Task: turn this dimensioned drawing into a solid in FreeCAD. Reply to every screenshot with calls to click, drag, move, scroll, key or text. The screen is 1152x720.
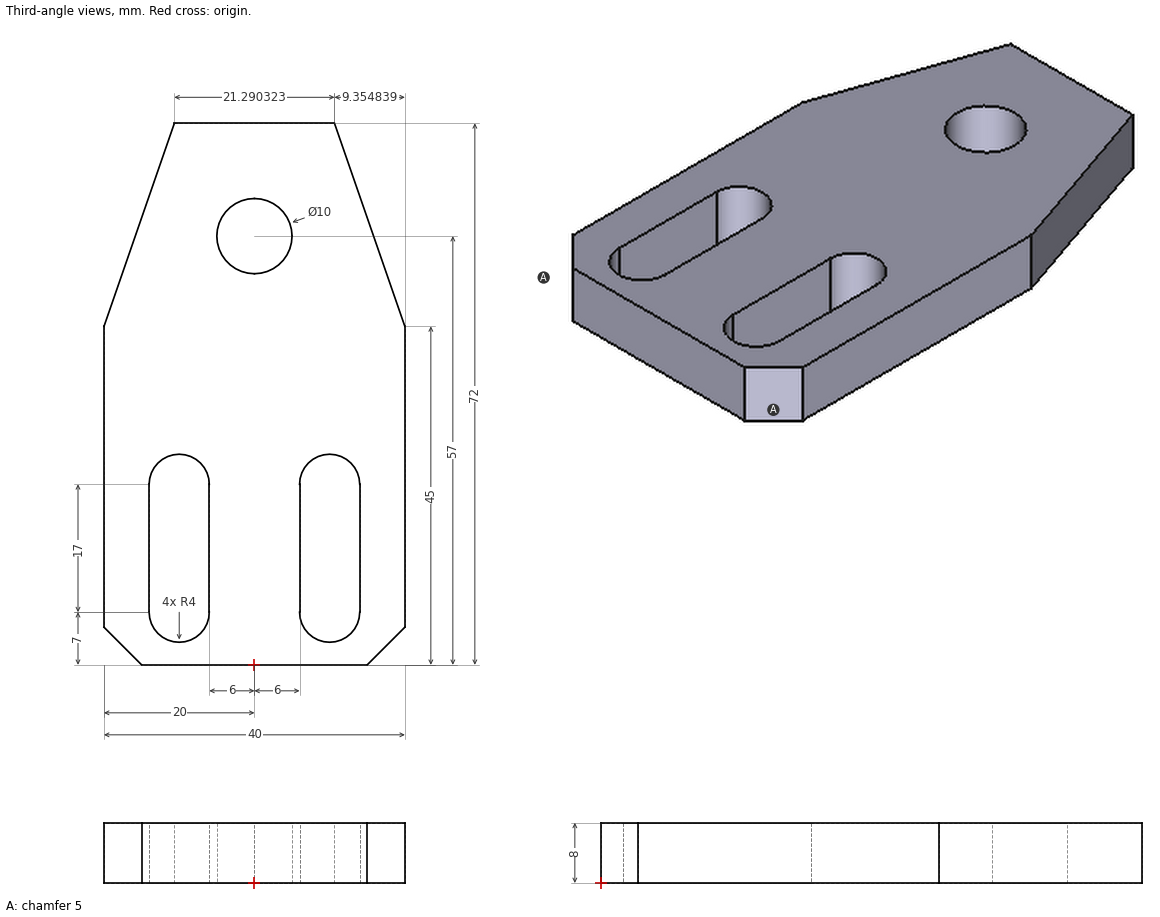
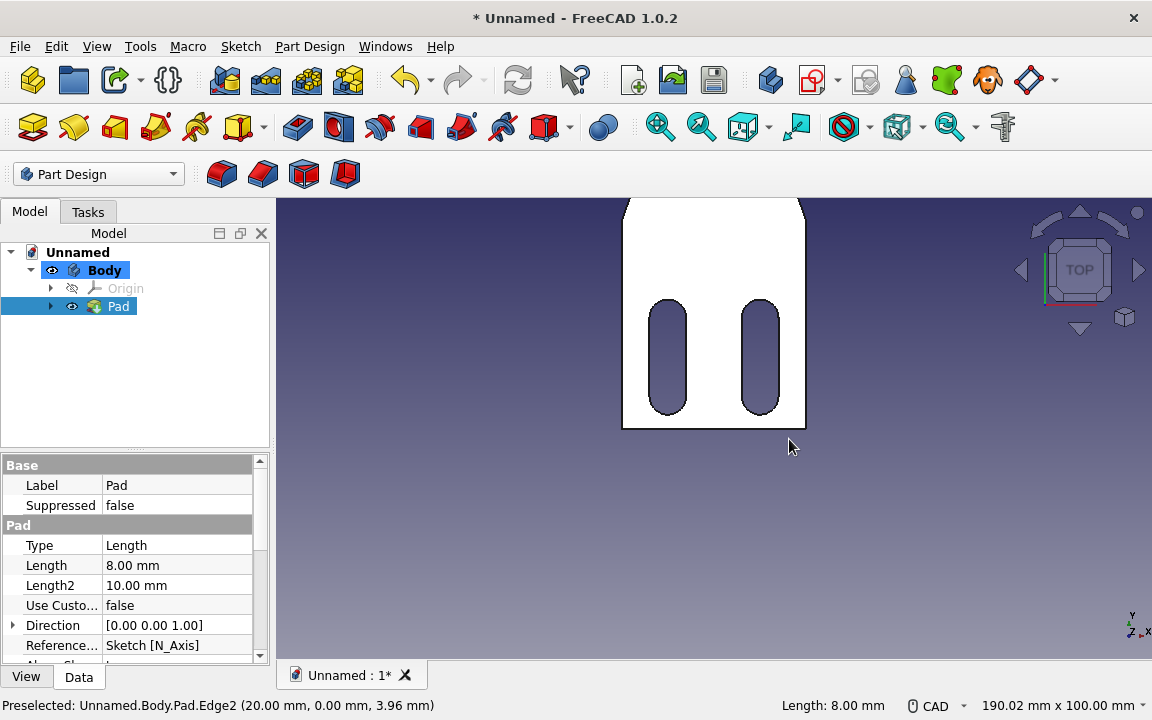
click(661, 128)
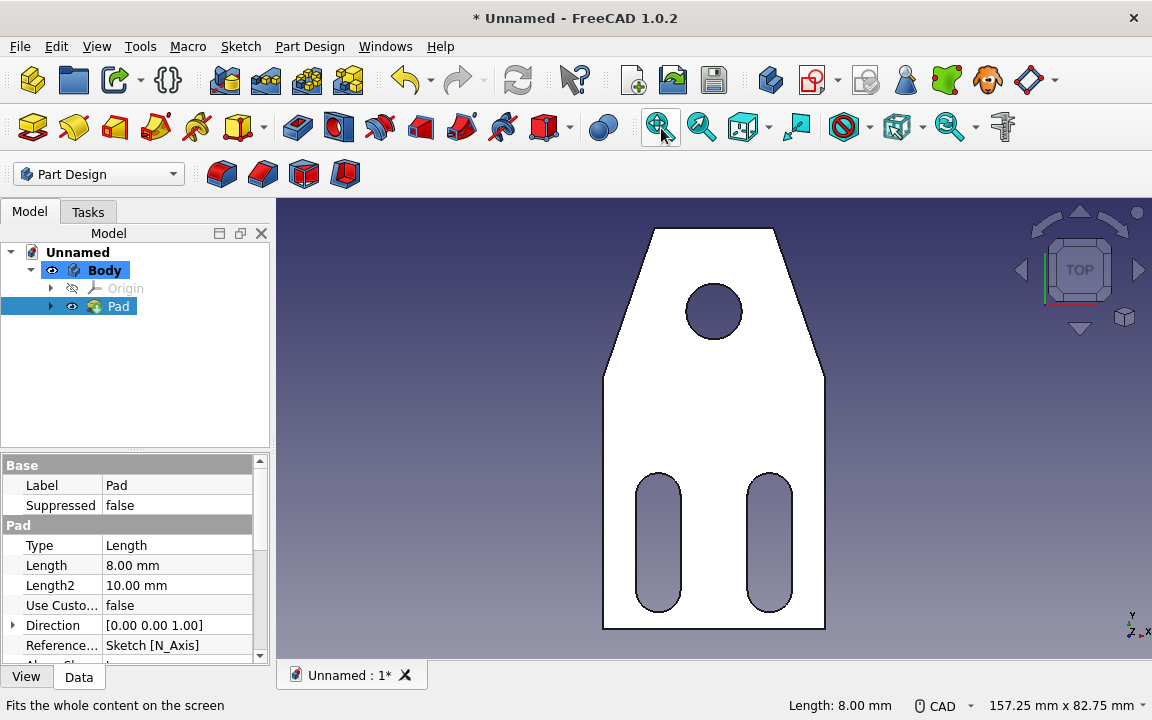
key(1)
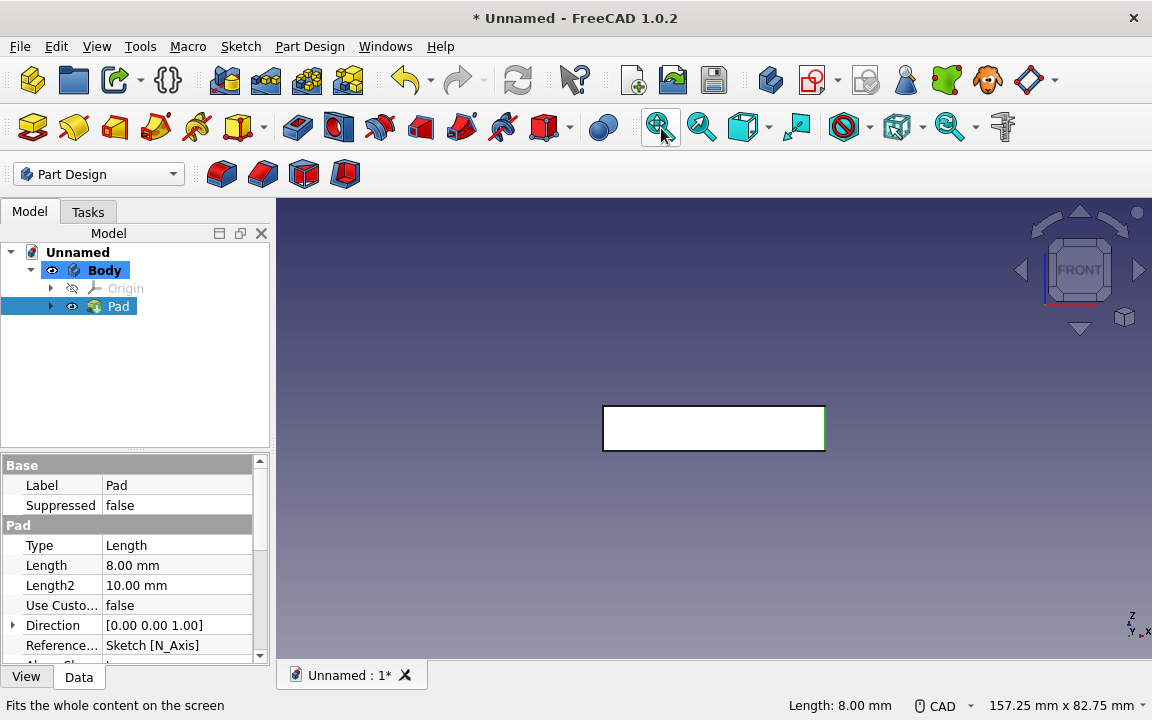
click(661, 128)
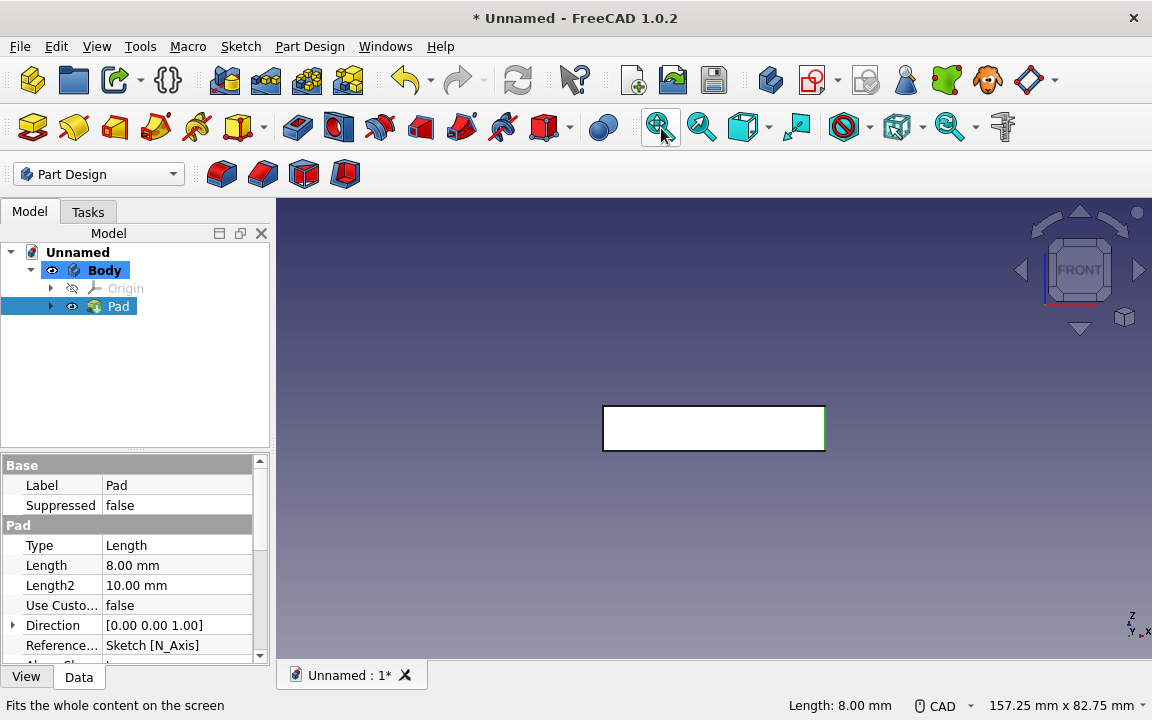
click(603, 428, ctrl)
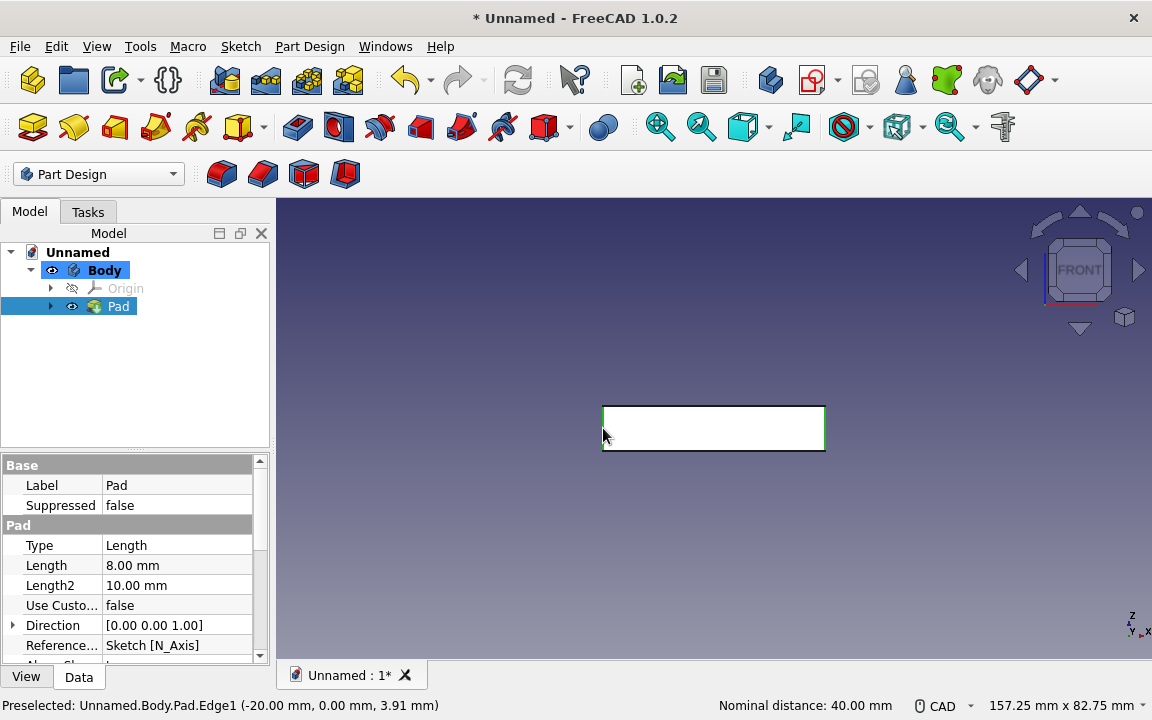
click(263, 174)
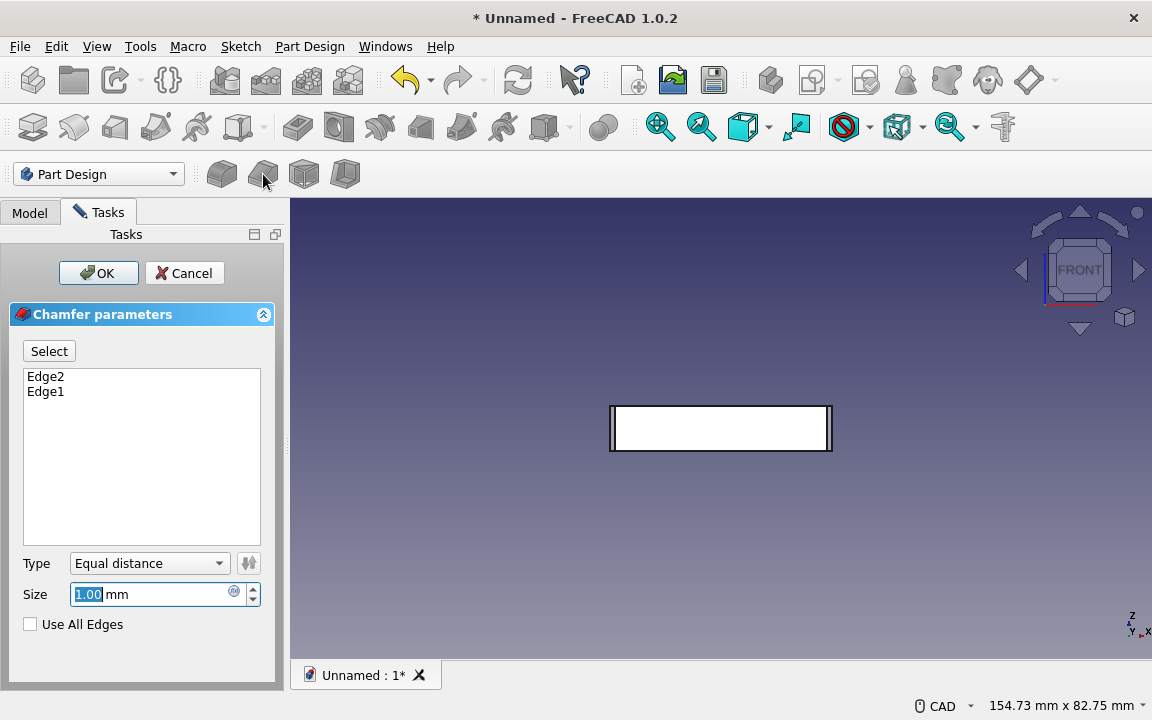
text(5)
key(Tab)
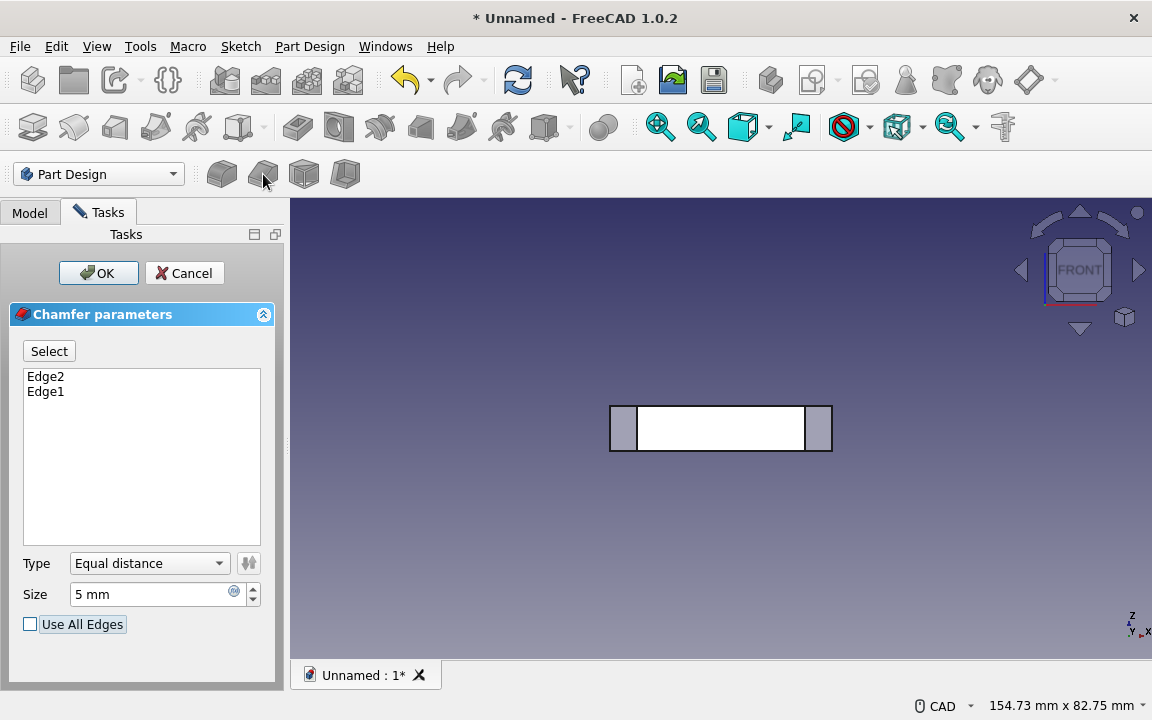
click(99, 273)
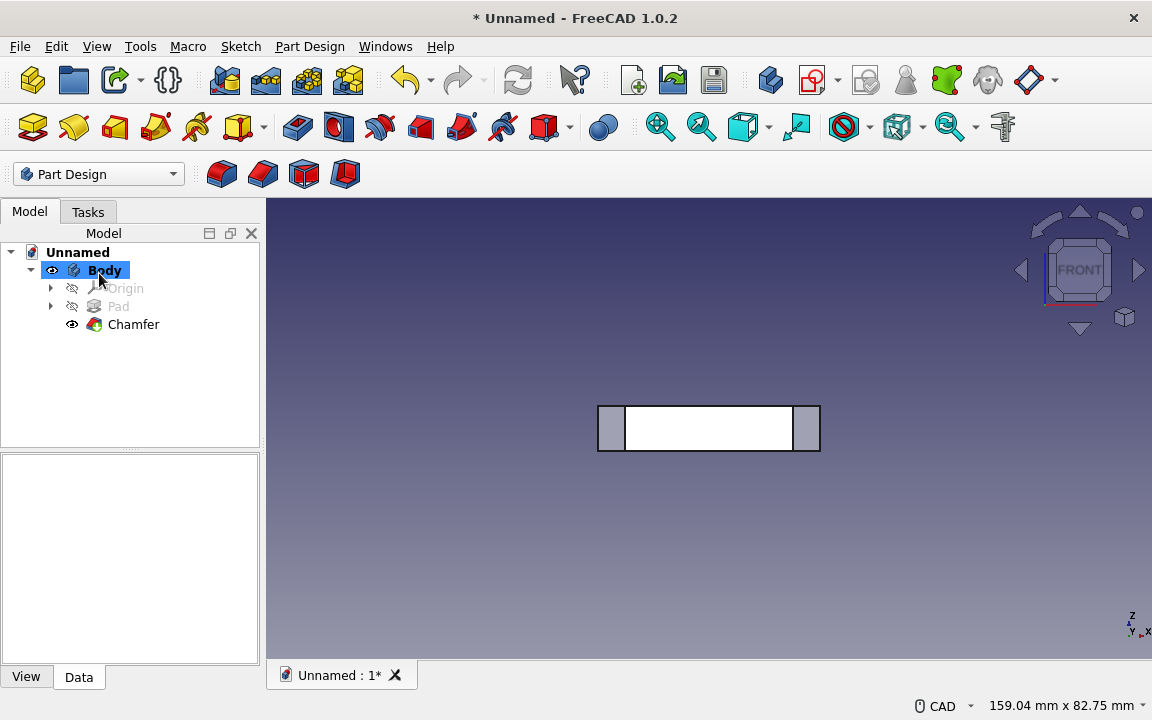
key(0)